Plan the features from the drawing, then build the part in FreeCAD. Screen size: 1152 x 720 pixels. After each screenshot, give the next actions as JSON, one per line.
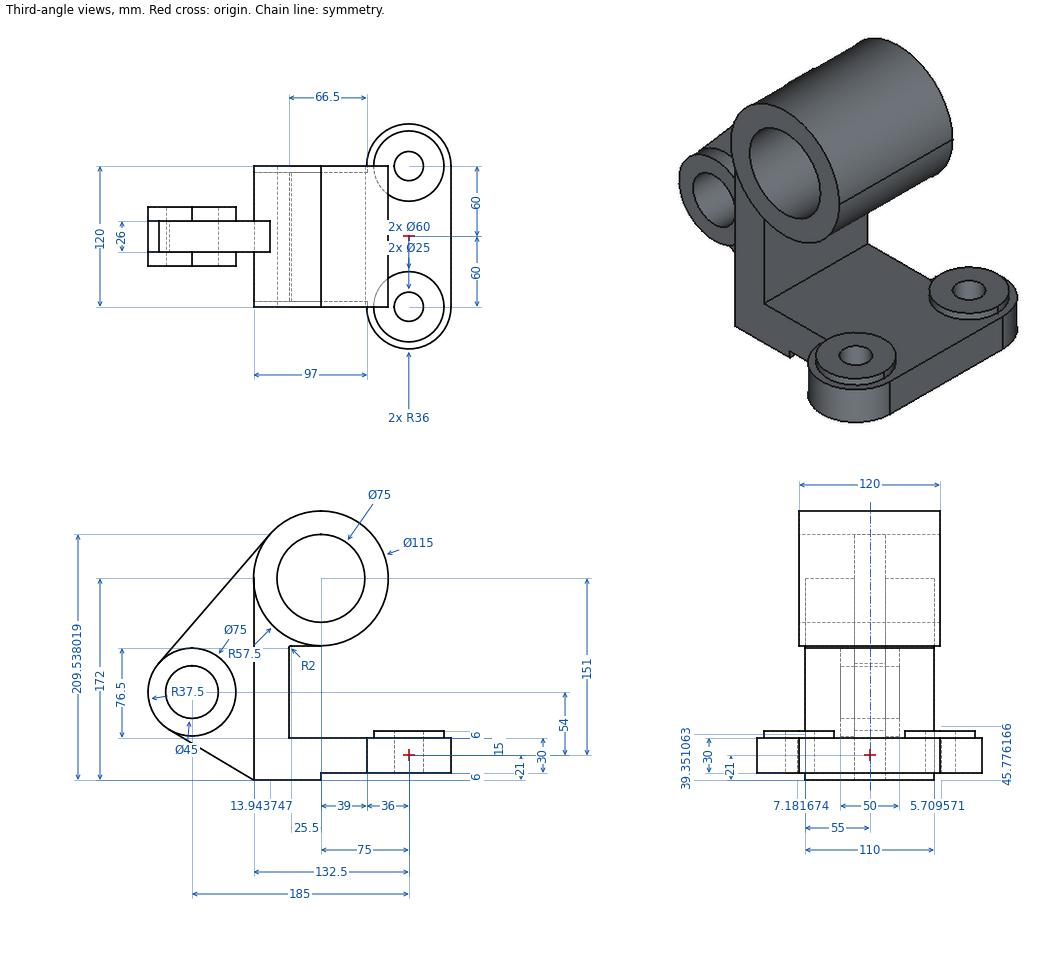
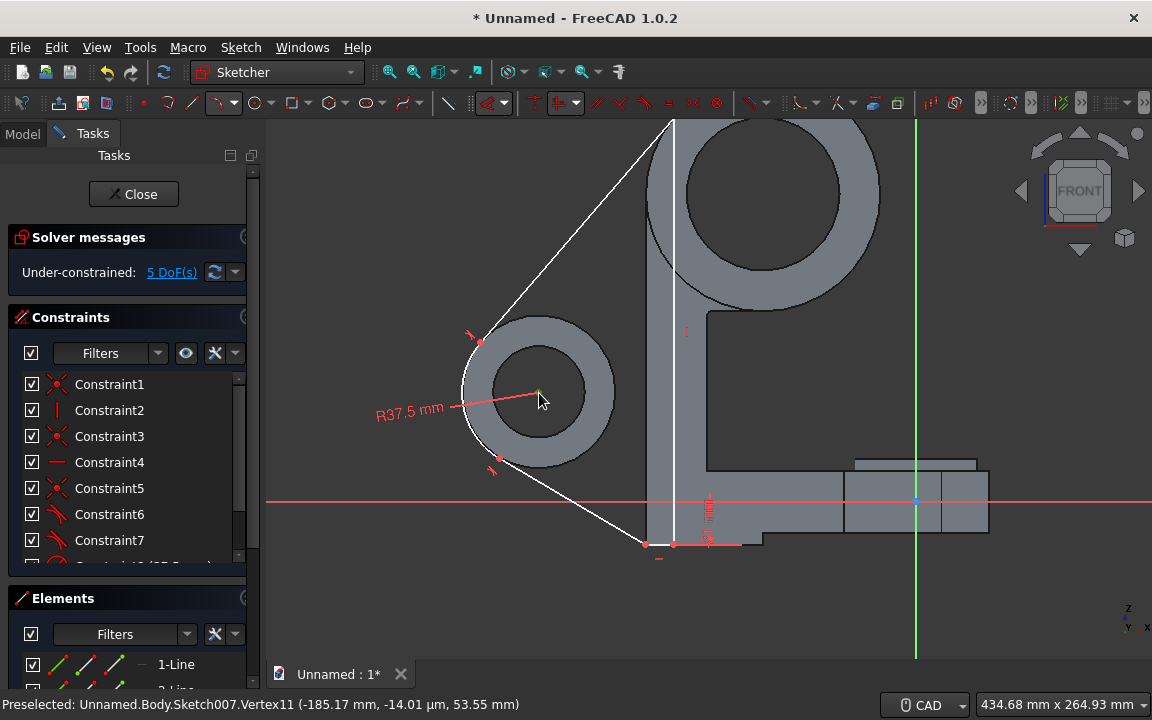
{"action": "key", "text": "i"}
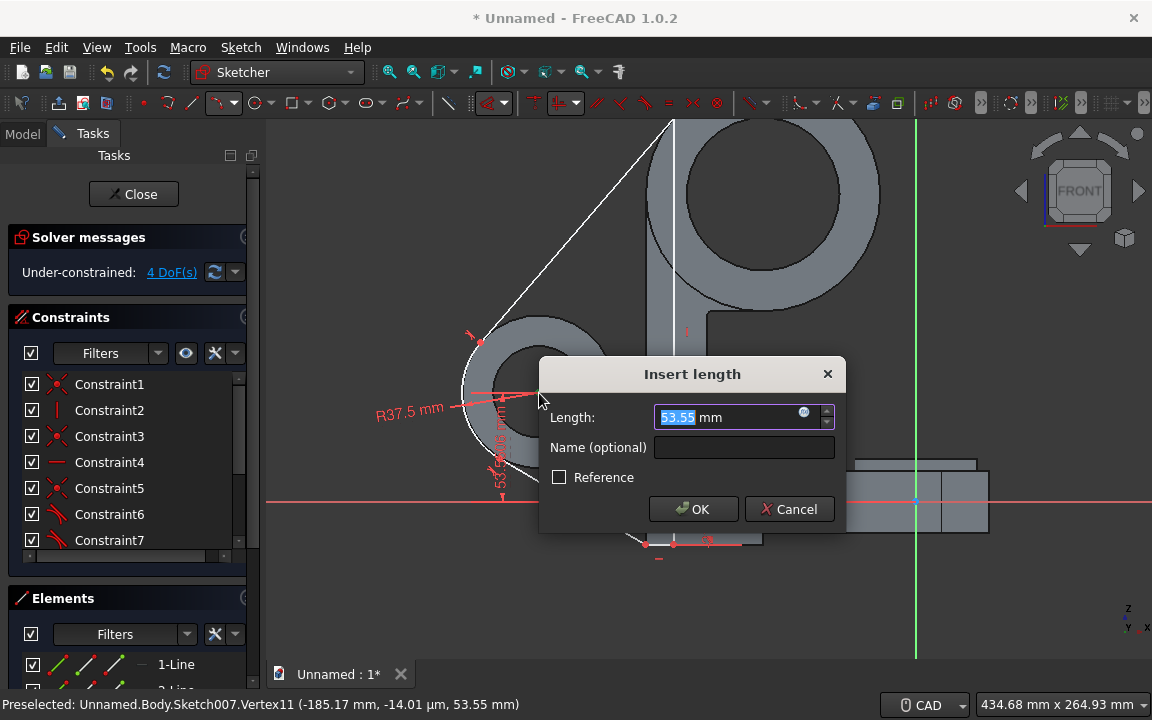
{"action": "type", "text": "54"}
{"action": "key", "text": "Return"}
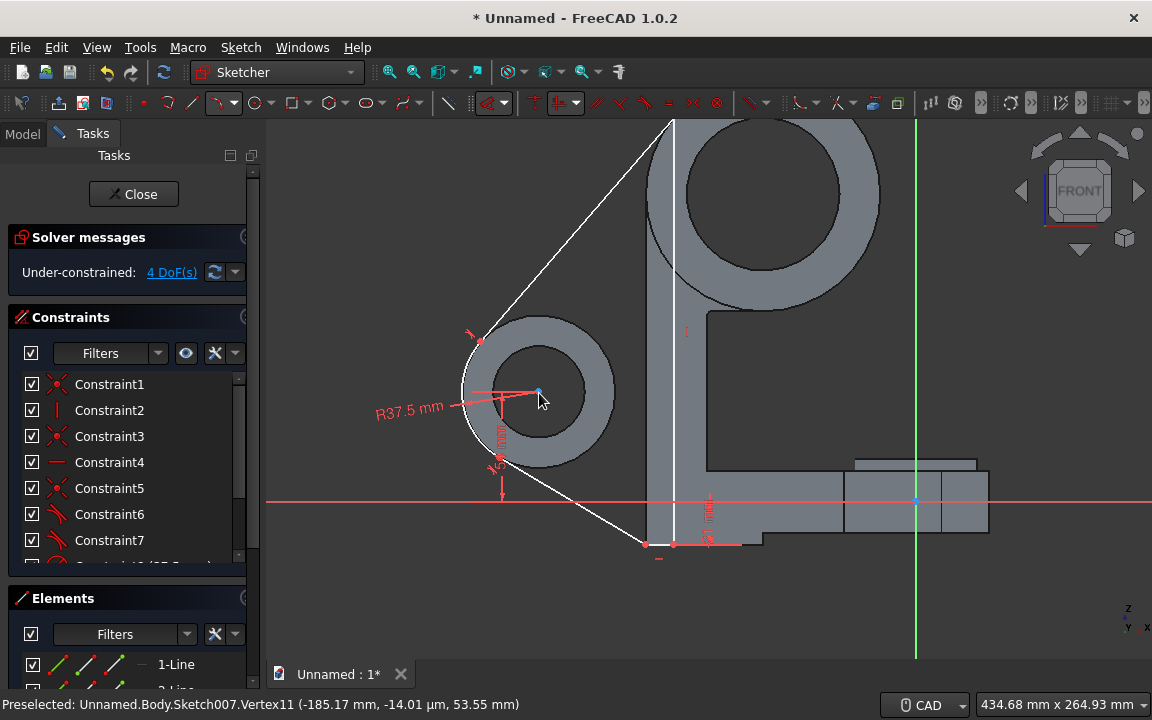
{"action": "left_click", "coordinate": [538, 392]}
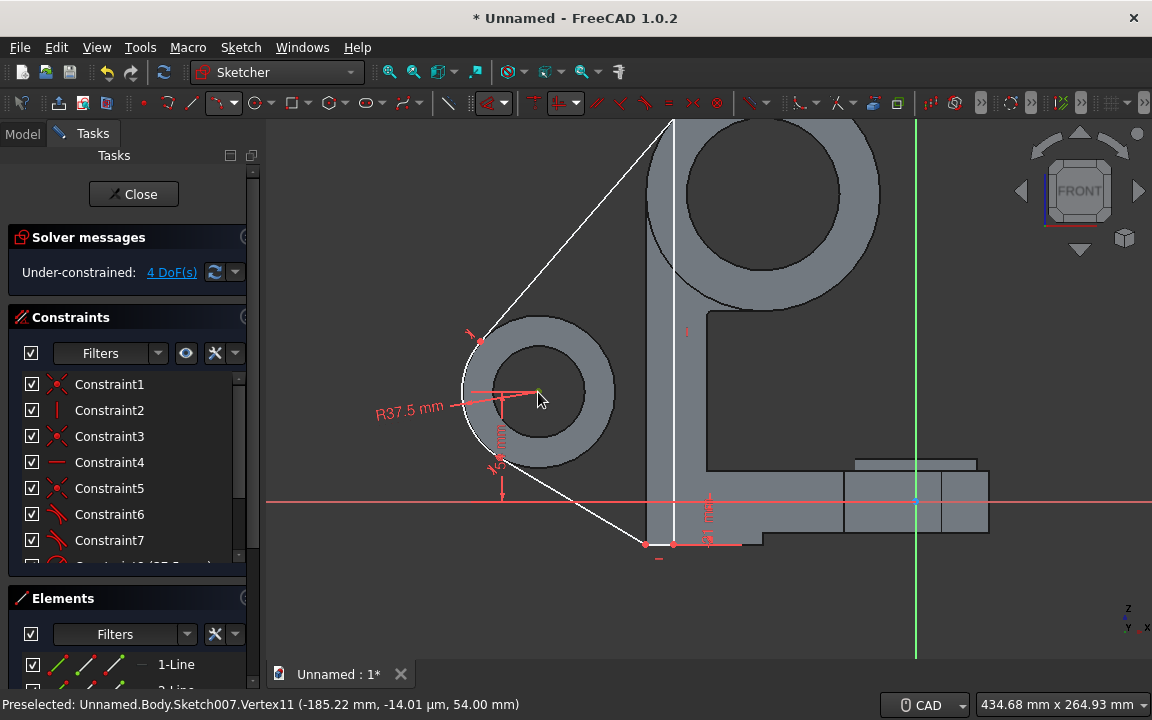
{"action": "key", "text": "l"}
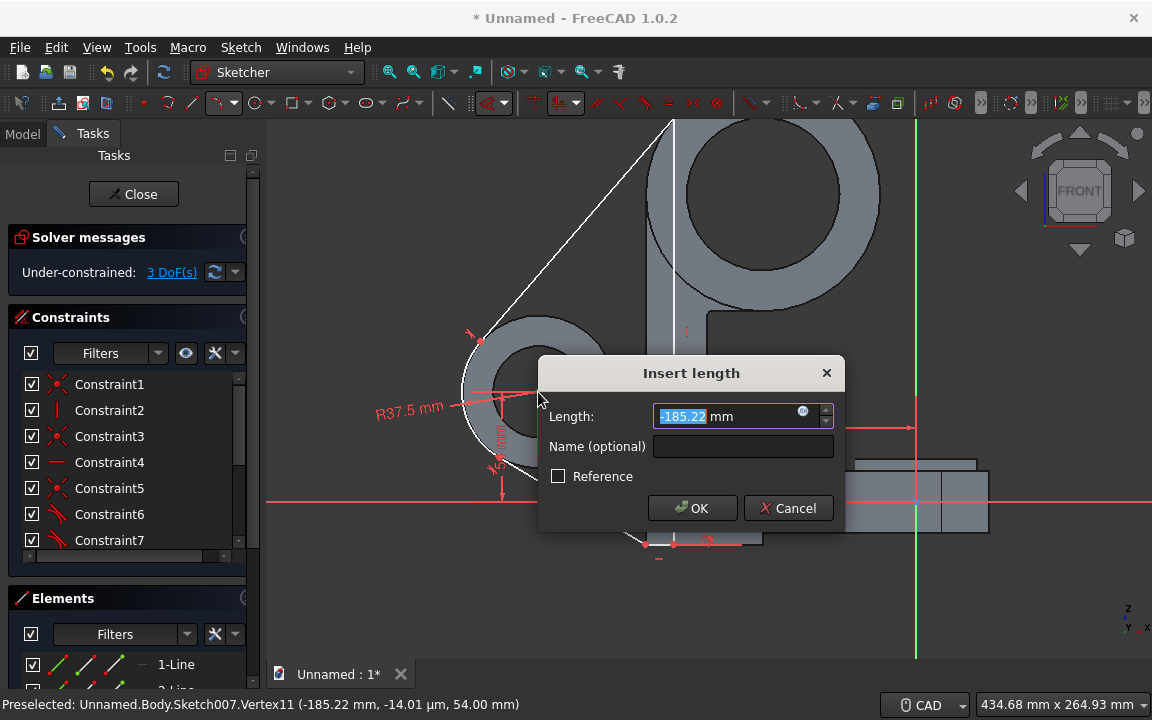
{"action": "type", "text": "-185"}
{"action": "key", "text": "Return"}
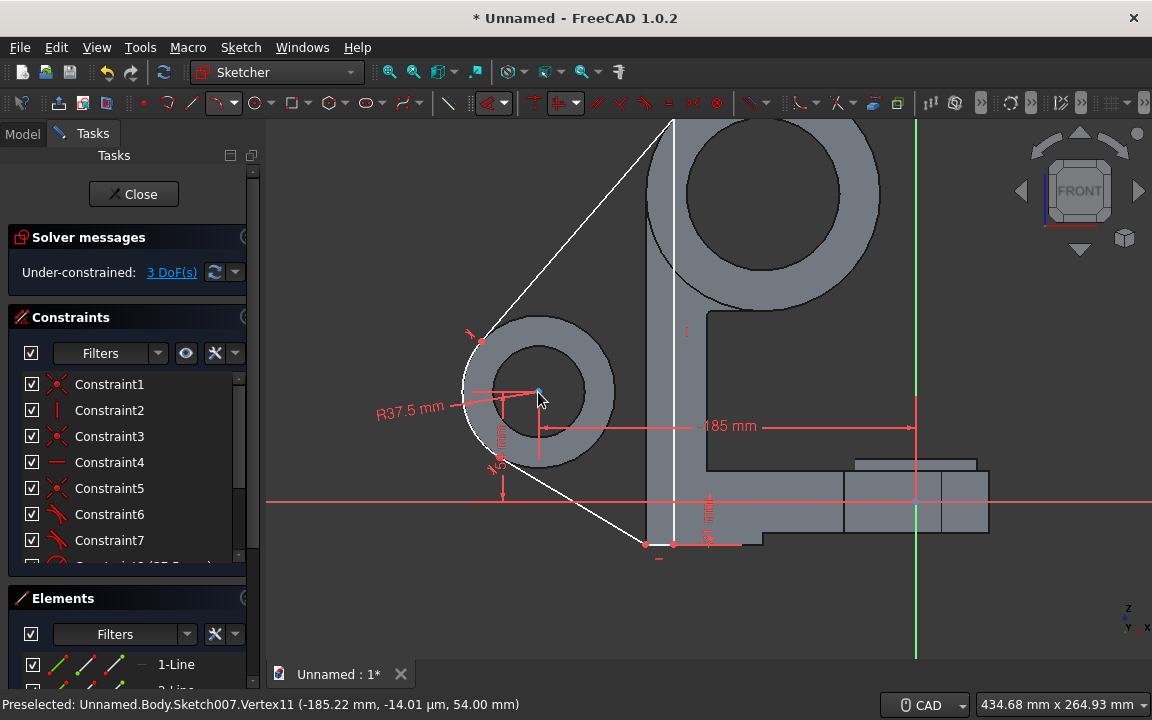
{"action": "left_click", "coordinate": [645, 545]}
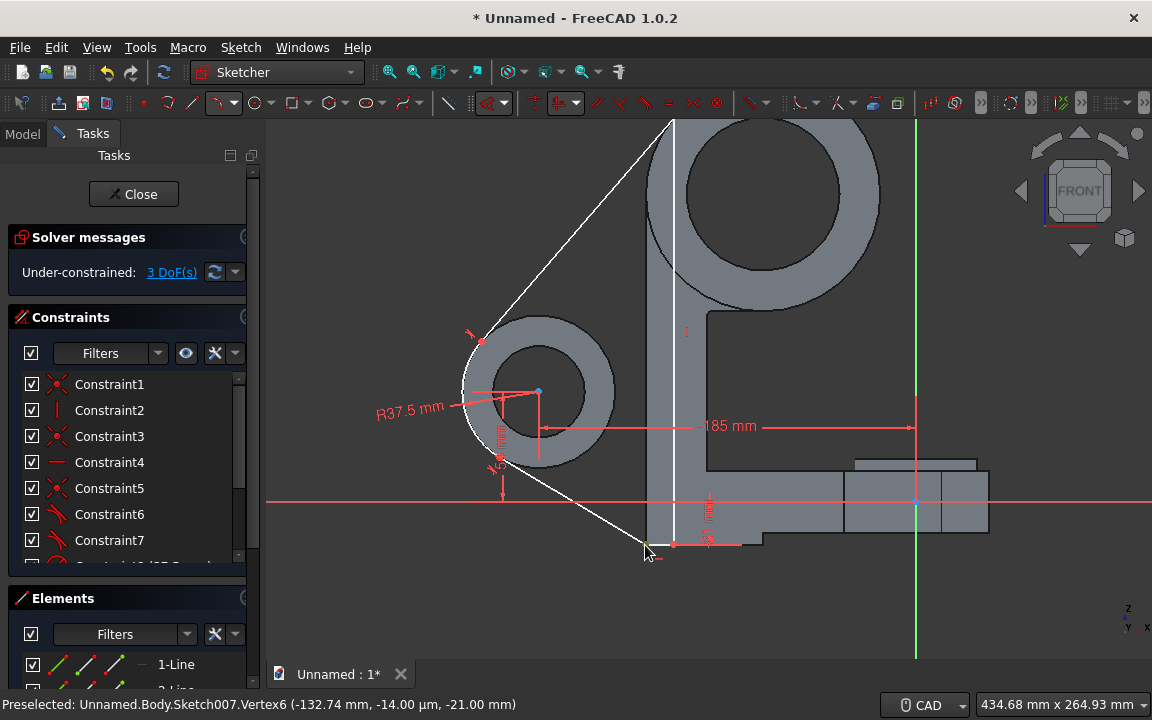
{"action": "key", "text": "l"}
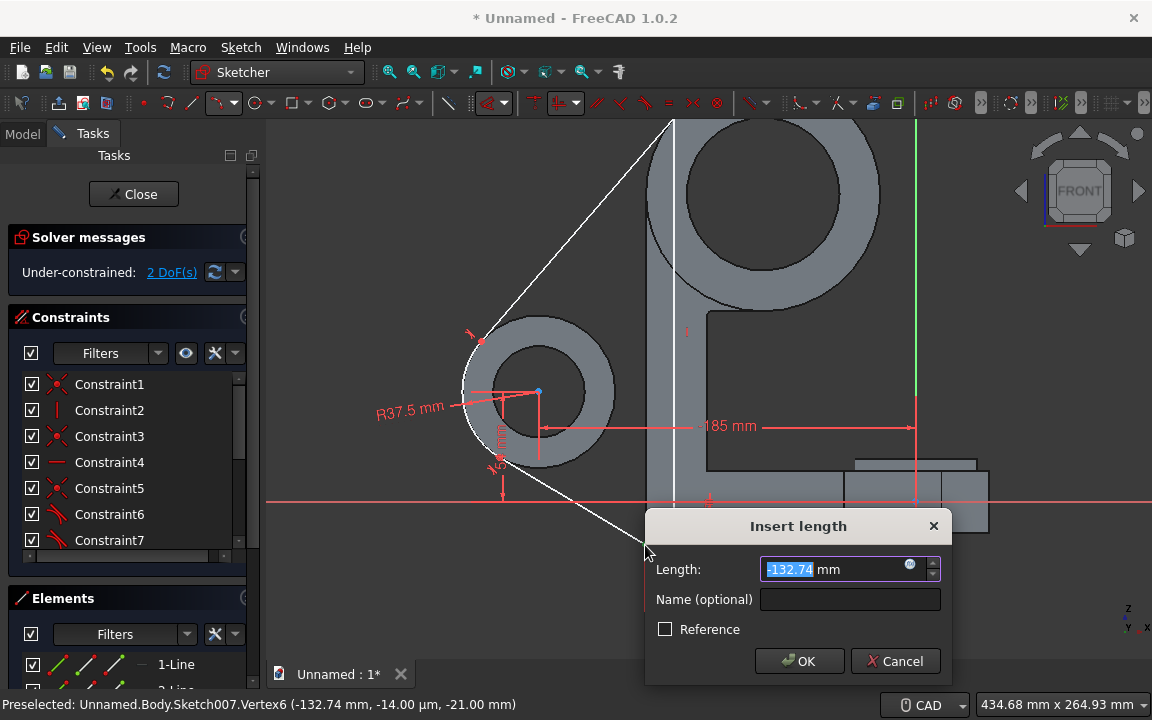
{"action": "type", "text": "-132.5"}
{"action": "key", "text": "Return"}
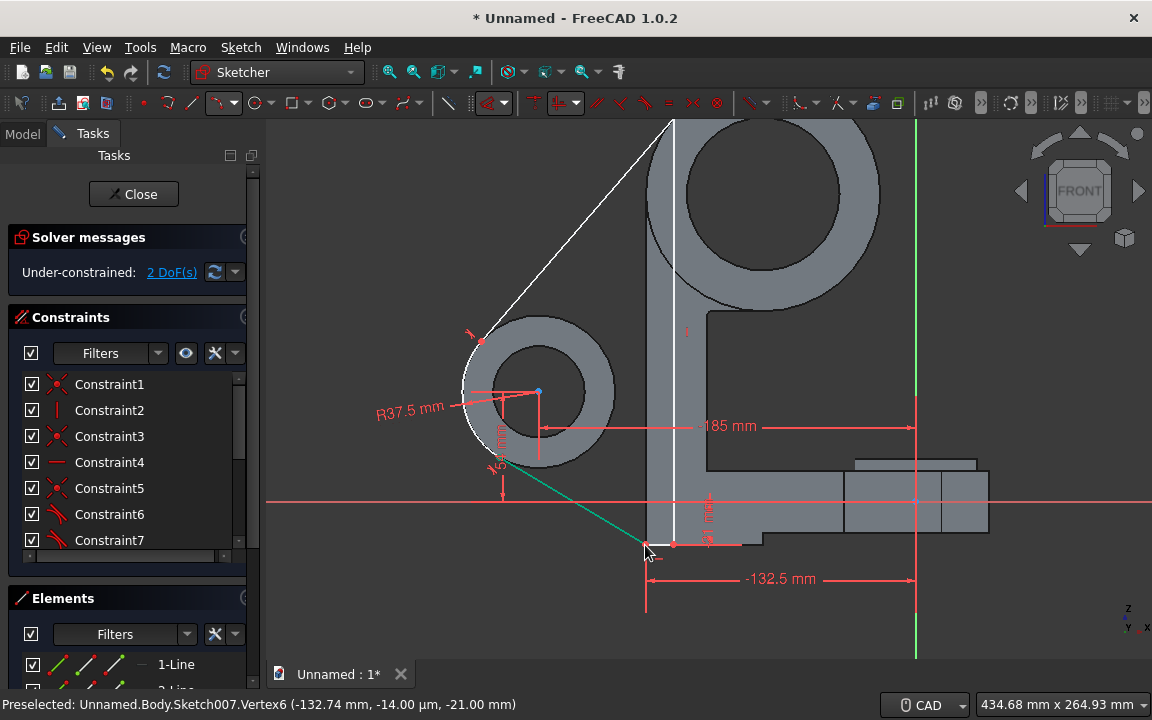
{"action": "scroll", "coordinate": [663, 545], "scroll_direction": "up", "scroll_amount": 2}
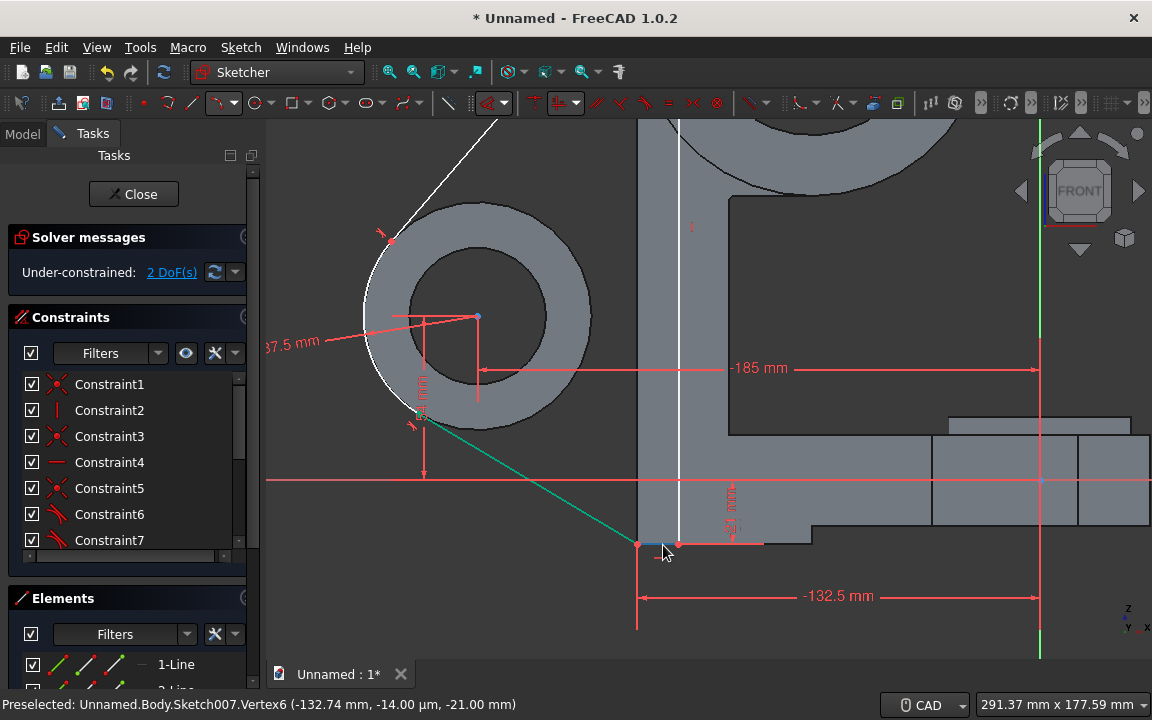
{"action": "left_click", "coordinate": [662, 544]}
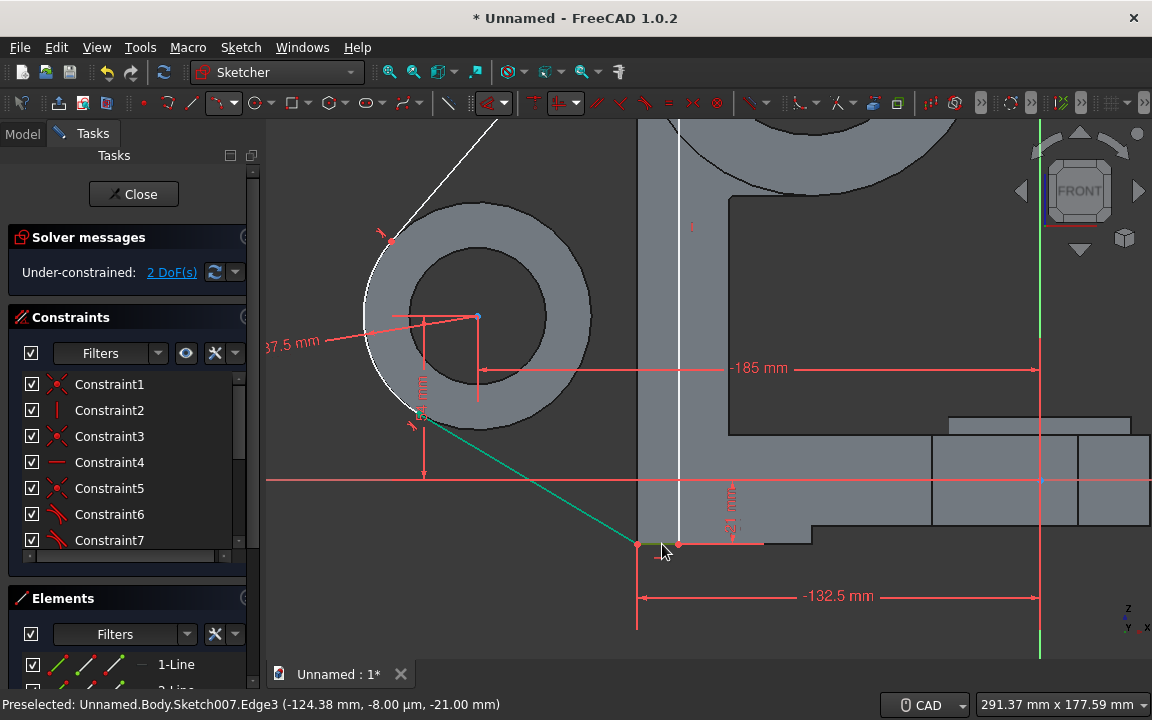
{"action": "key", "text": "l"}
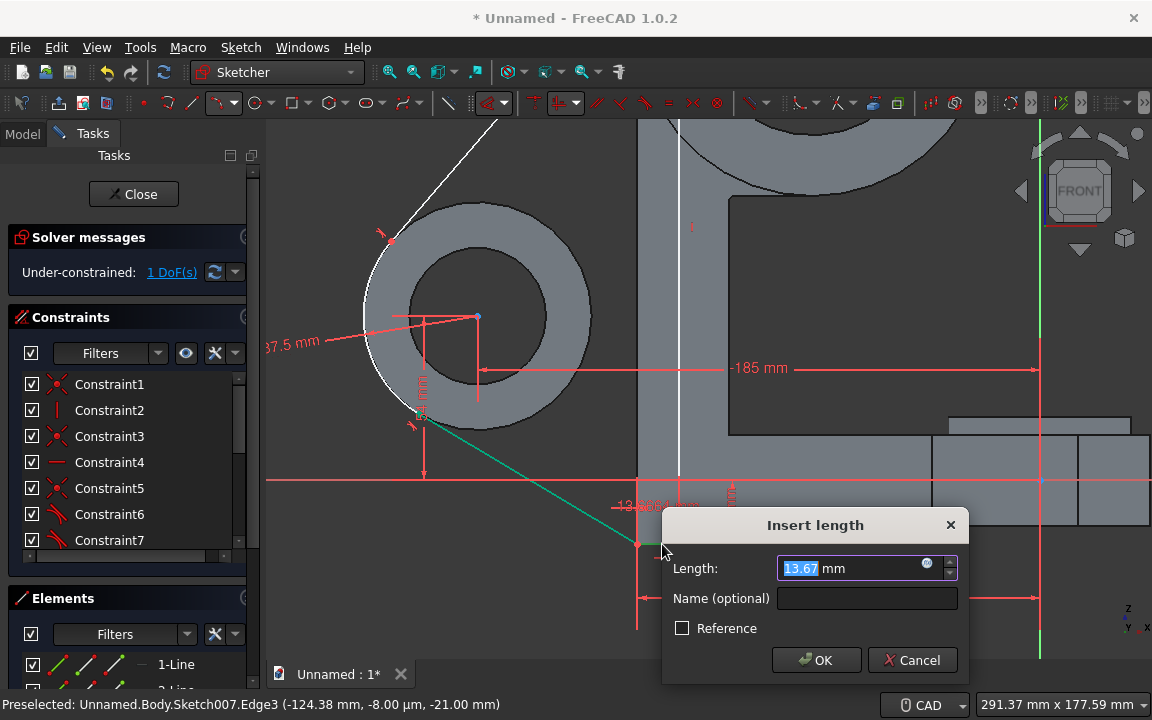
{"action": "type", "text": "13.943747"}
{"action": "key", "text": "Return"}